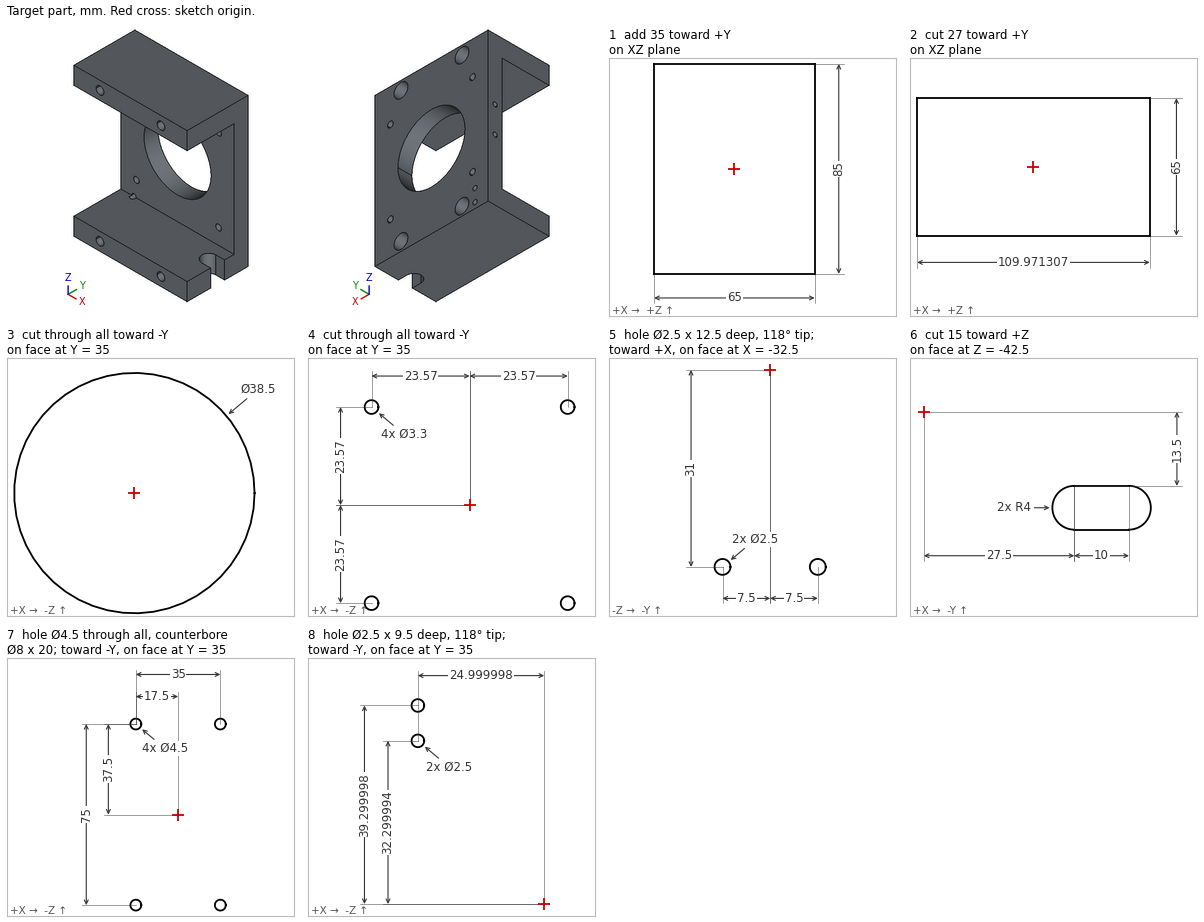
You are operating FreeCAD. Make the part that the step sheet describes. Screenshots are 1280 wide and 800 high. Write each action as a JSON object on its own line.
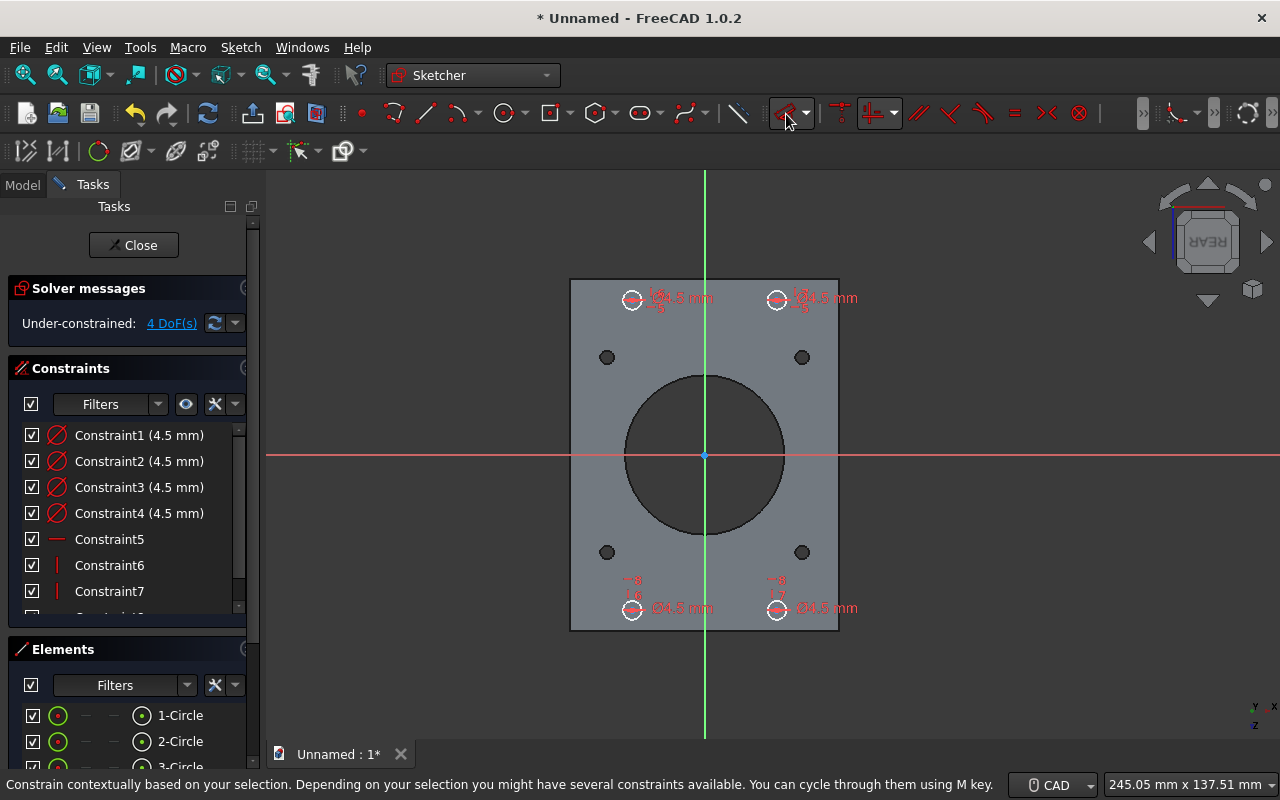
{"action": "left_click", "coordinate": [632, 300]}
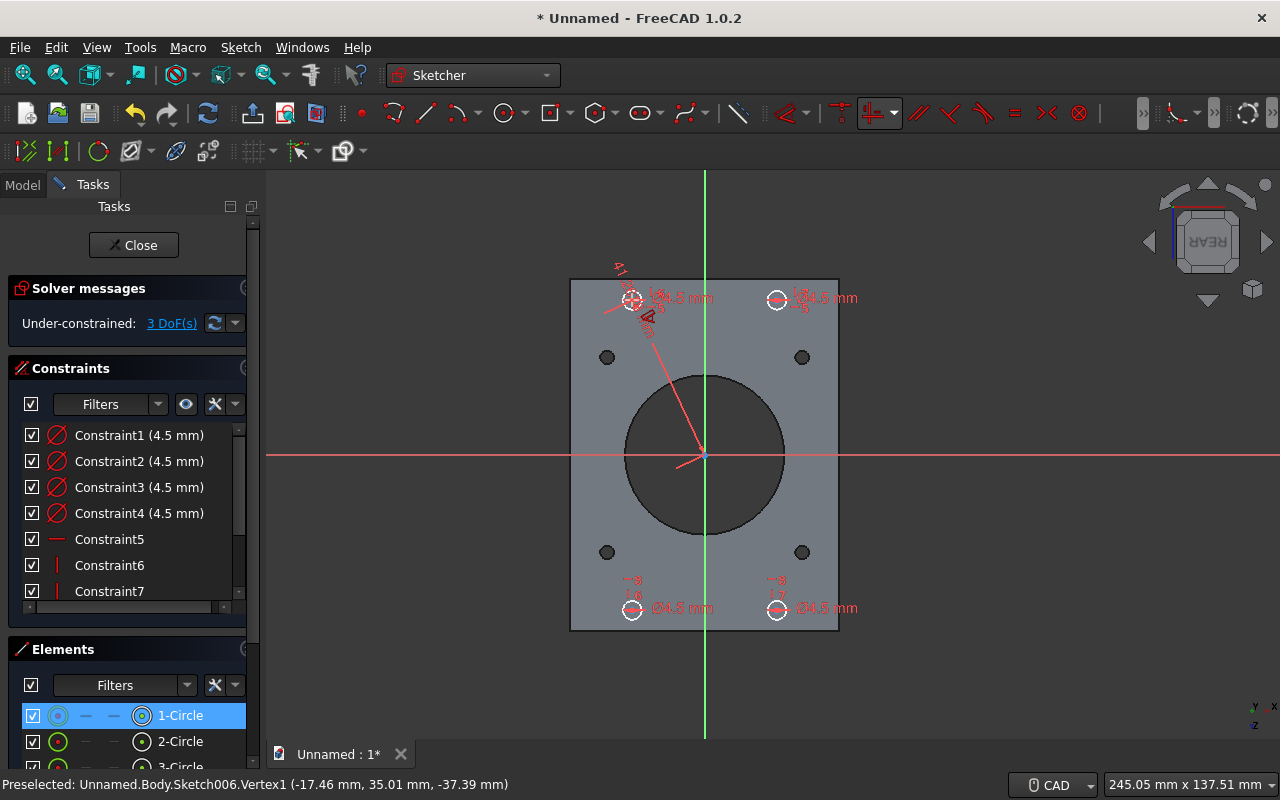
{"action": "left_click", "coordinate": [777, 300]}
{"action": "left_click", "coordinate": [671, 266]}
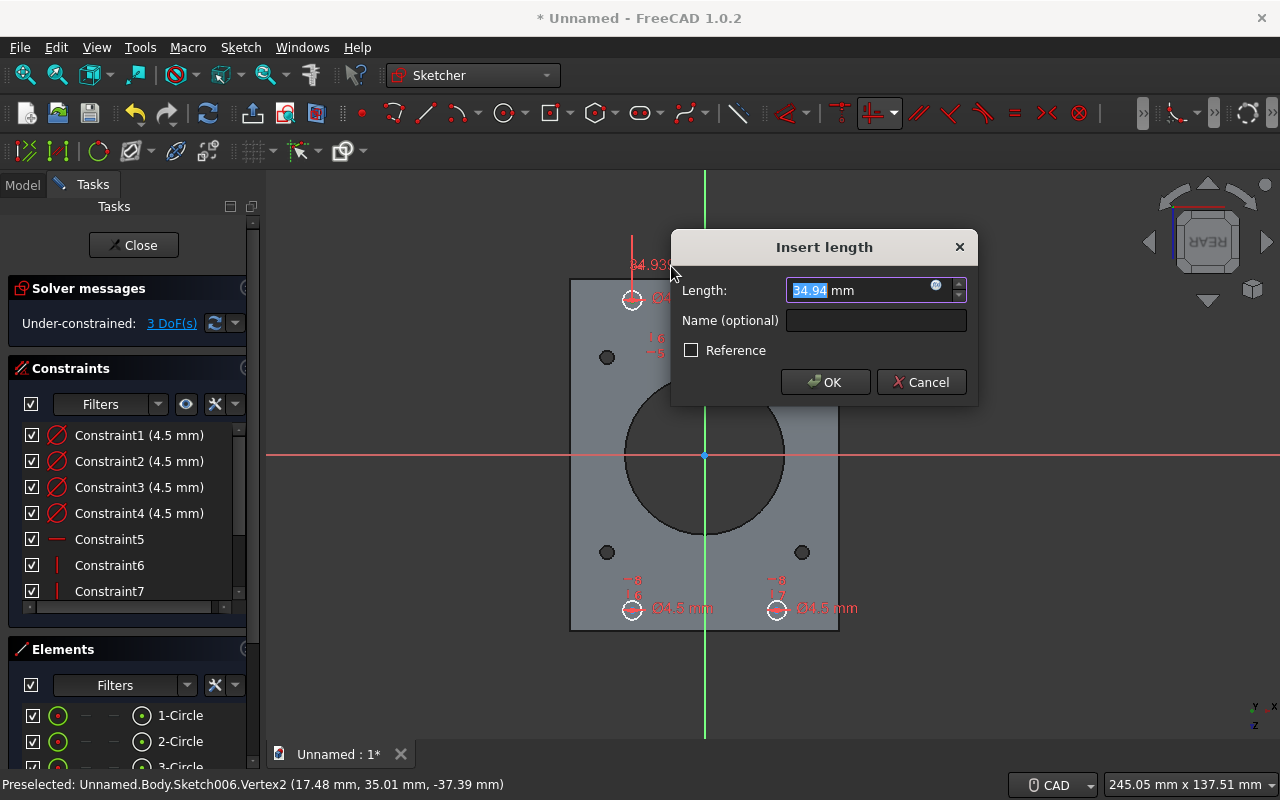
{"action": "type", "text": "35"}
{"action": "key", "text": "Return"}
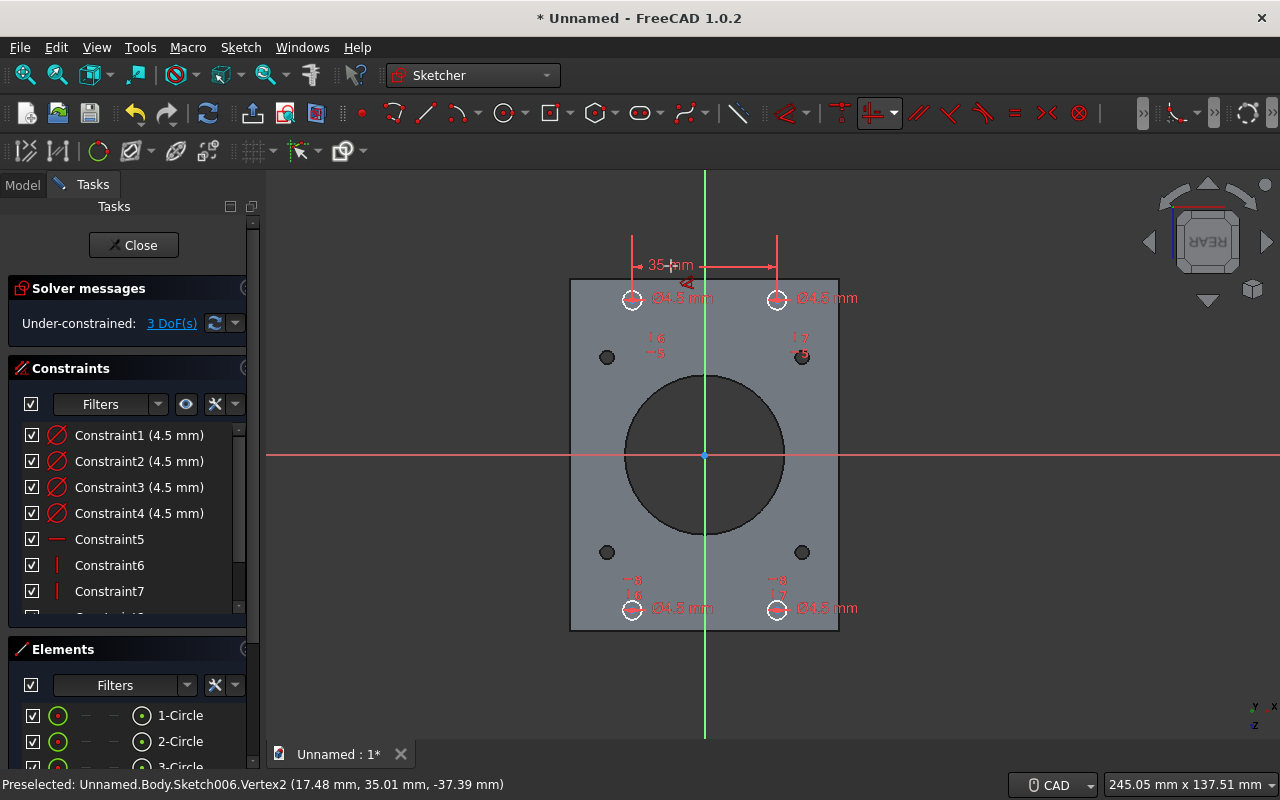
{"action": "left_click", "coordinate": [632, 300]}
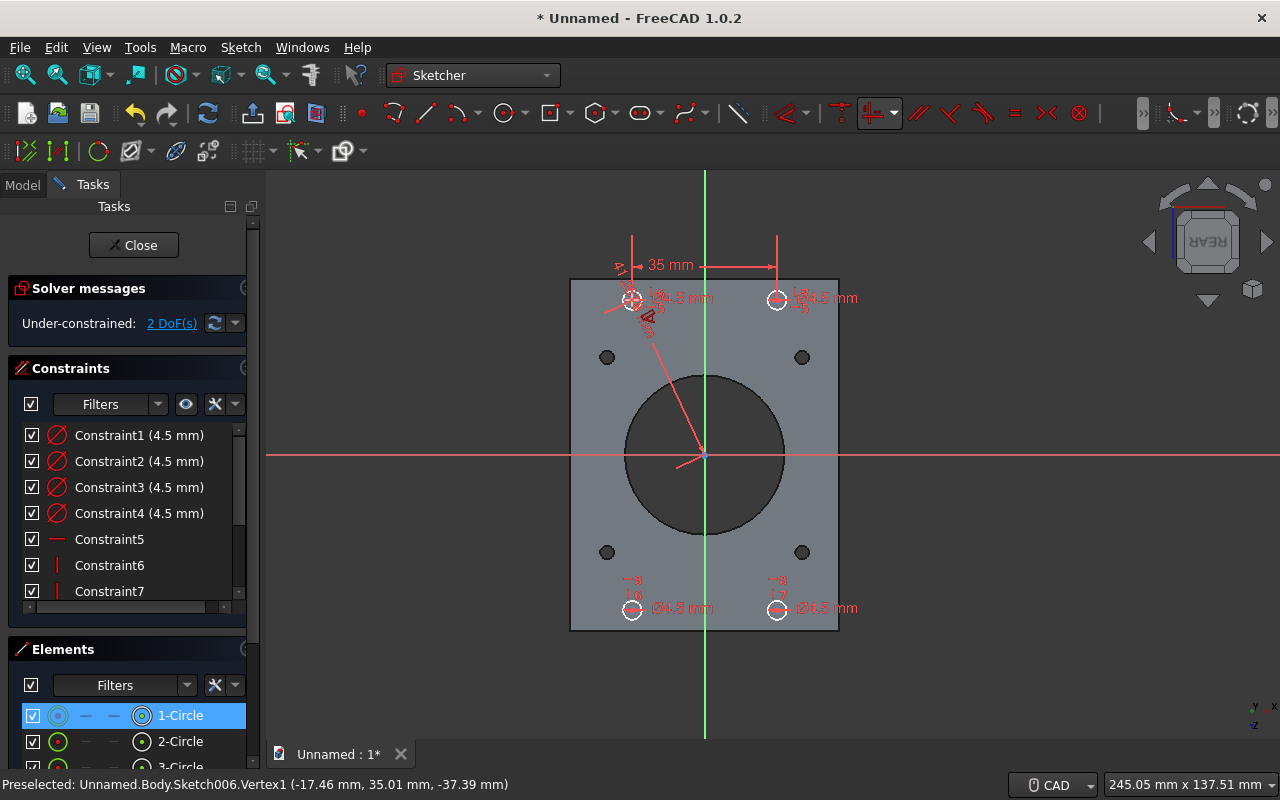
{"action": "left_click", "coordinate": [632, 610]}
{"action": "left_click", "coordinate": [598, 384]}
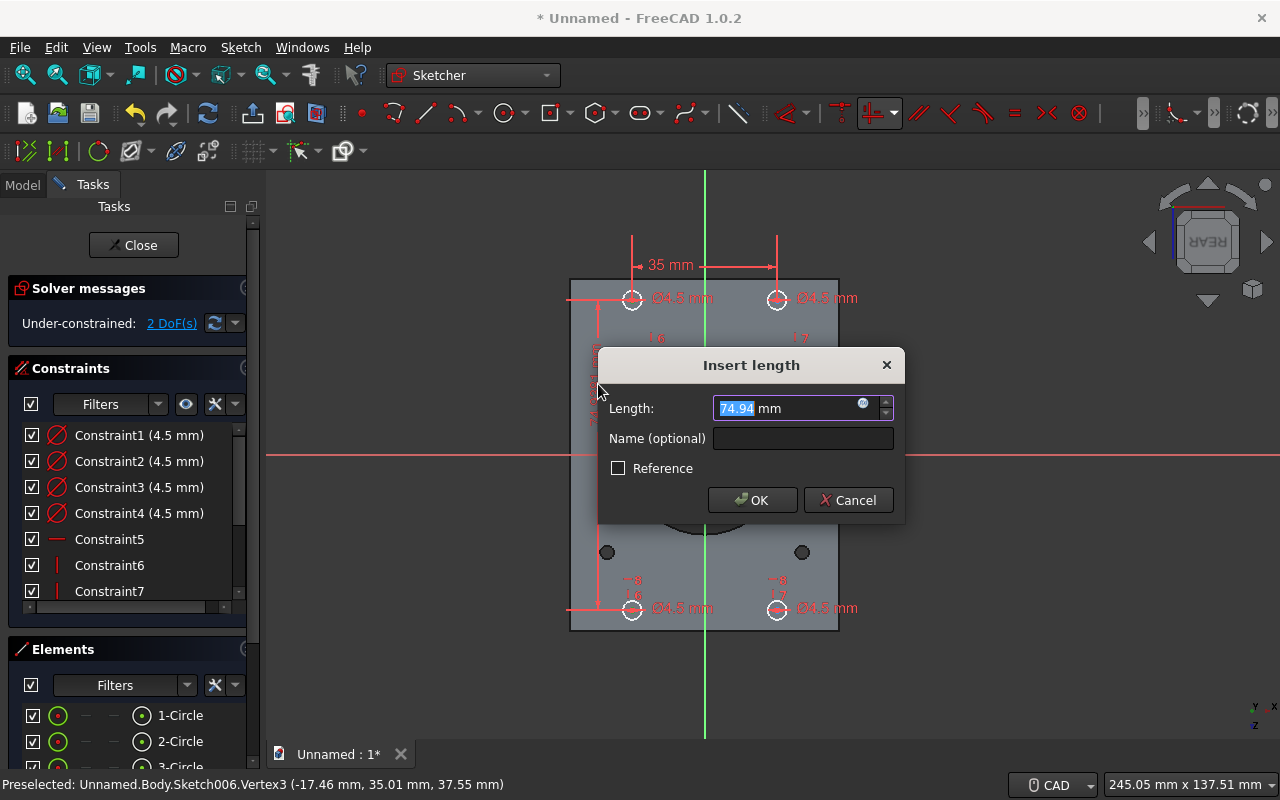
{"action": "type", "text": "75"}
{"action": "key", "text": "Return"}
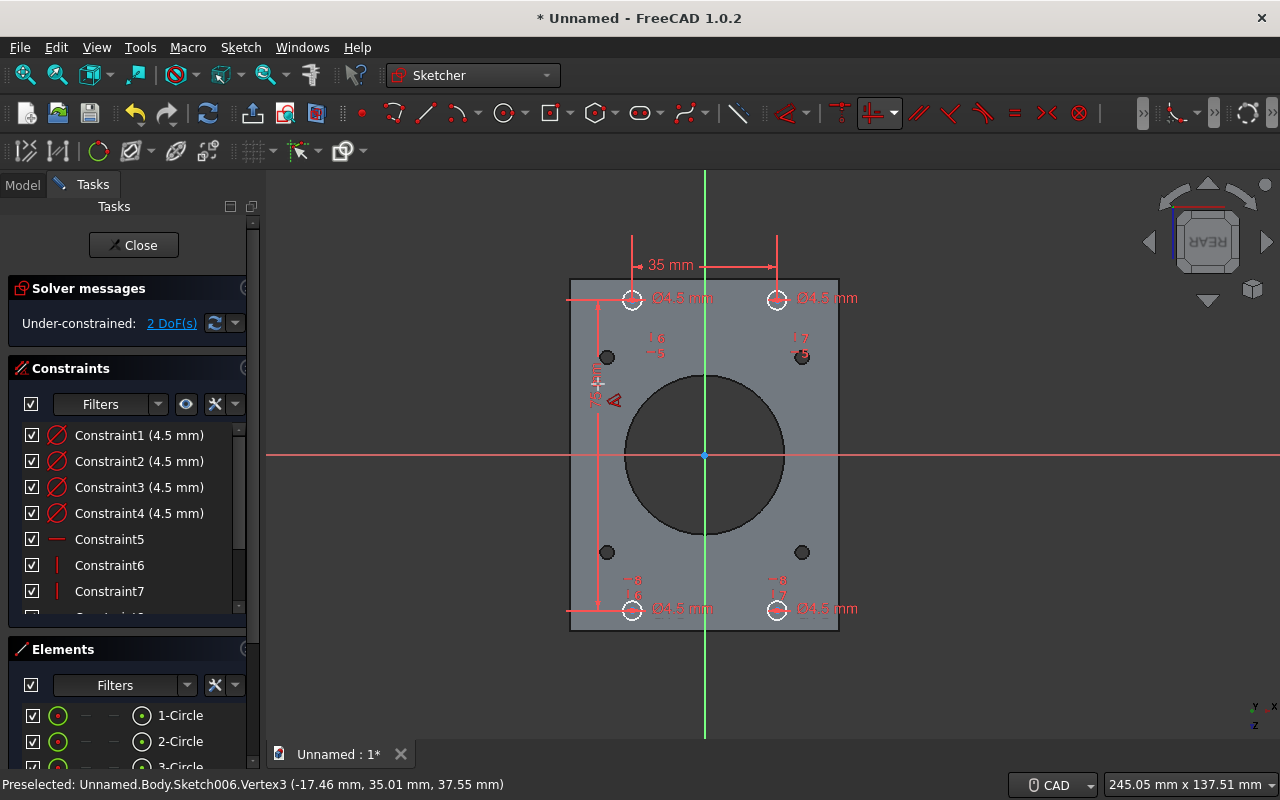
{"action": "left_click", "coordinate": [632, 300]}
{"action": "left_click", "coordinate": [668, 489]}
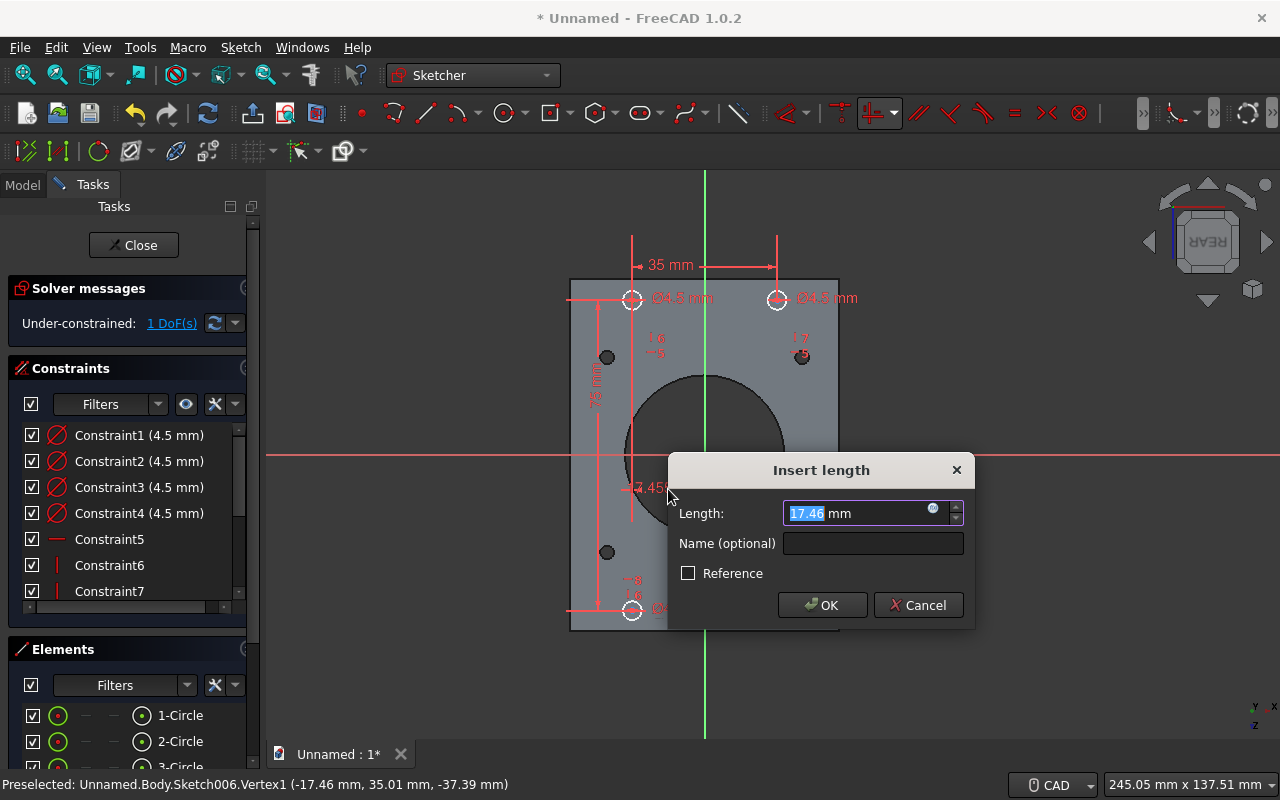
{"action": "type", "text": "17.5"}
{"action": "key", "text": "Return"}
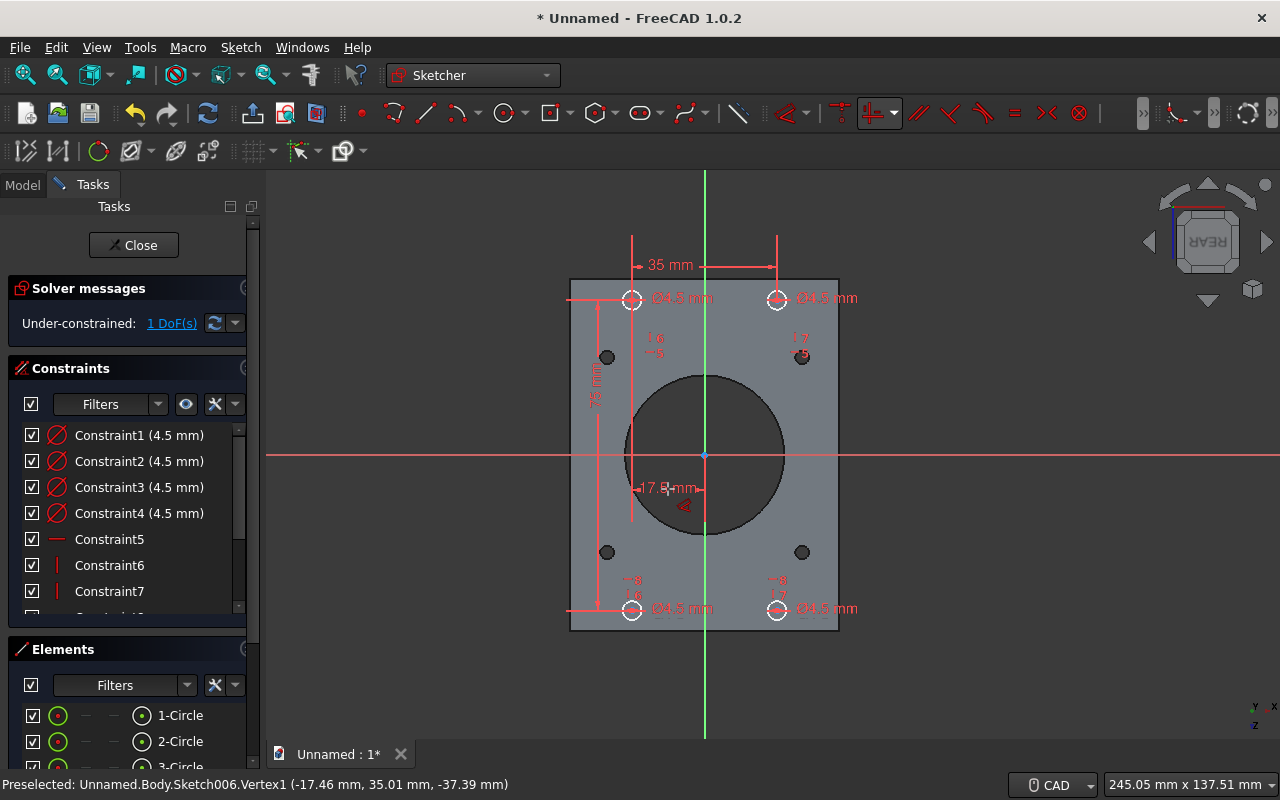
{"action": "left_click", "coordinate": [632, 300]}
{"action": "left_click", "coordinate": [598, 342]}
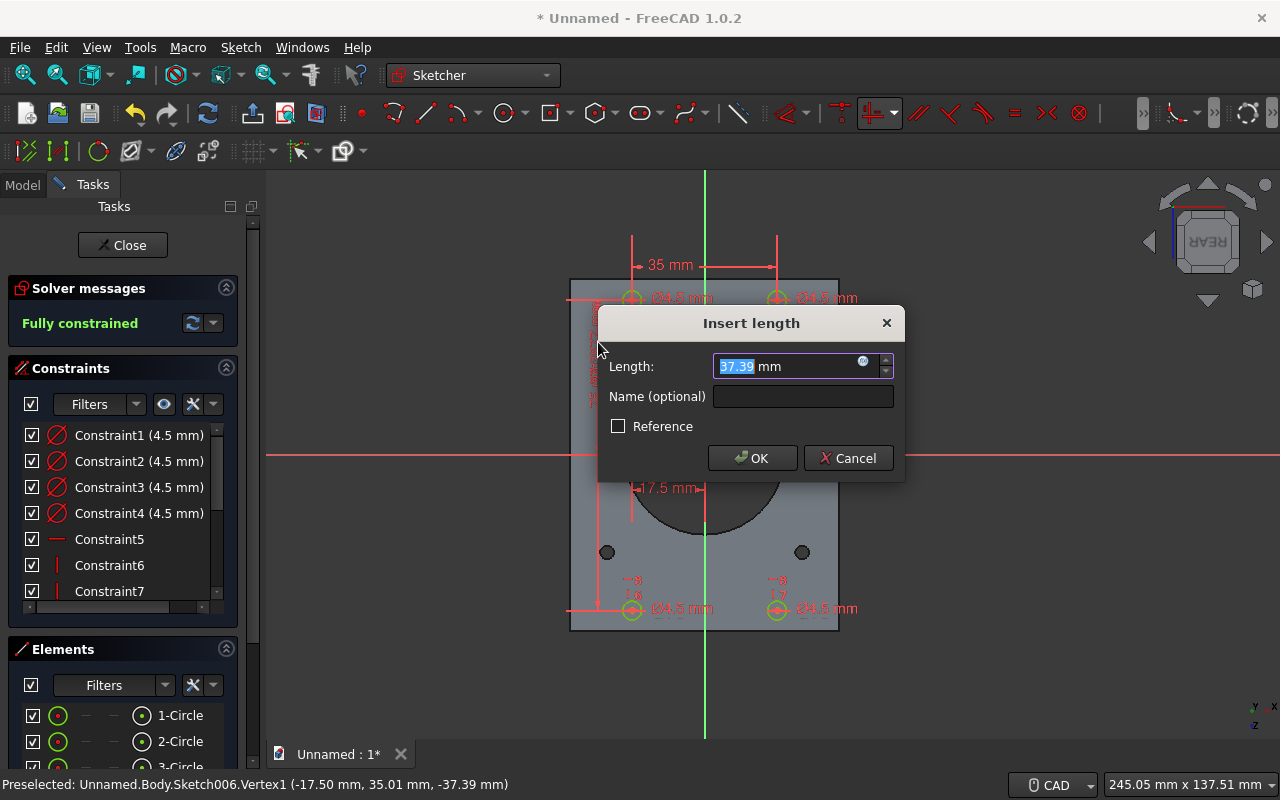
{"action": "type", "text": "37.5"}
{"action": "key", "text": "Return"}
{"action": "key", "text": "Escape"}